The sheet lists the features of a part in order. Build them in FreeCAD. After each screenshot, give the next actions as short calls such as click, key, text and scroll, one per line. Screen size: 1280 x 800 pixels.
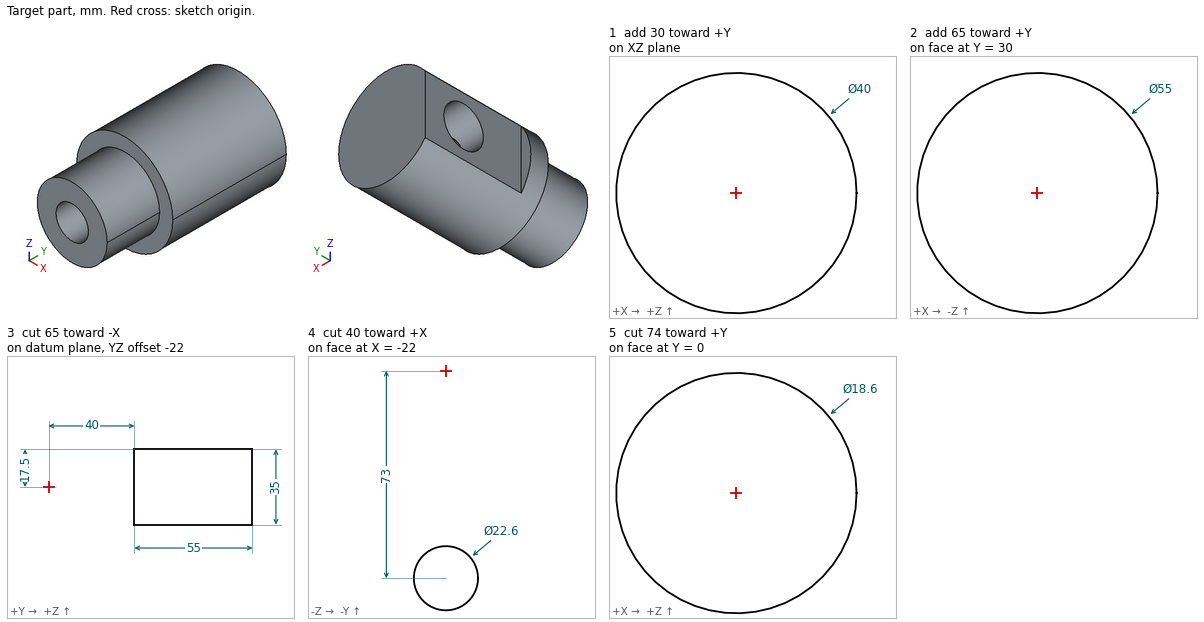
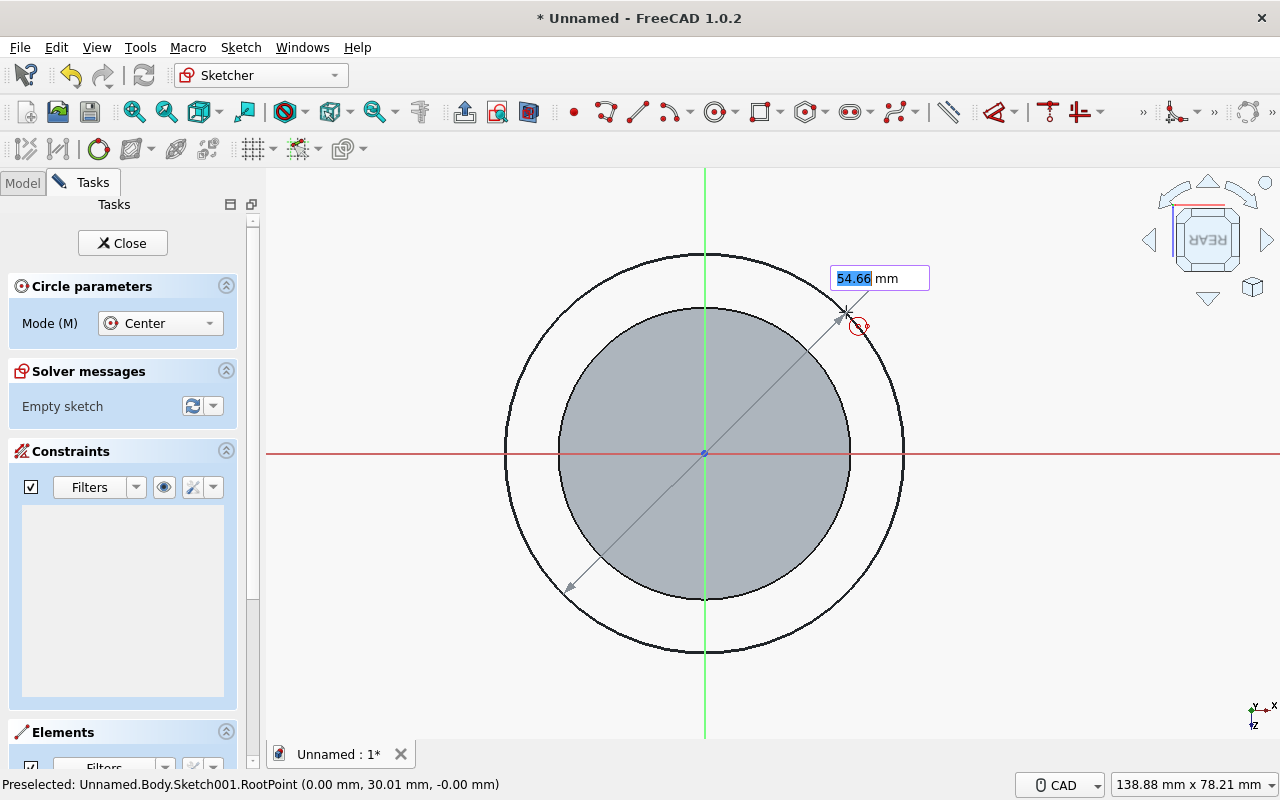
text(55)
key(Return)
key(Escape)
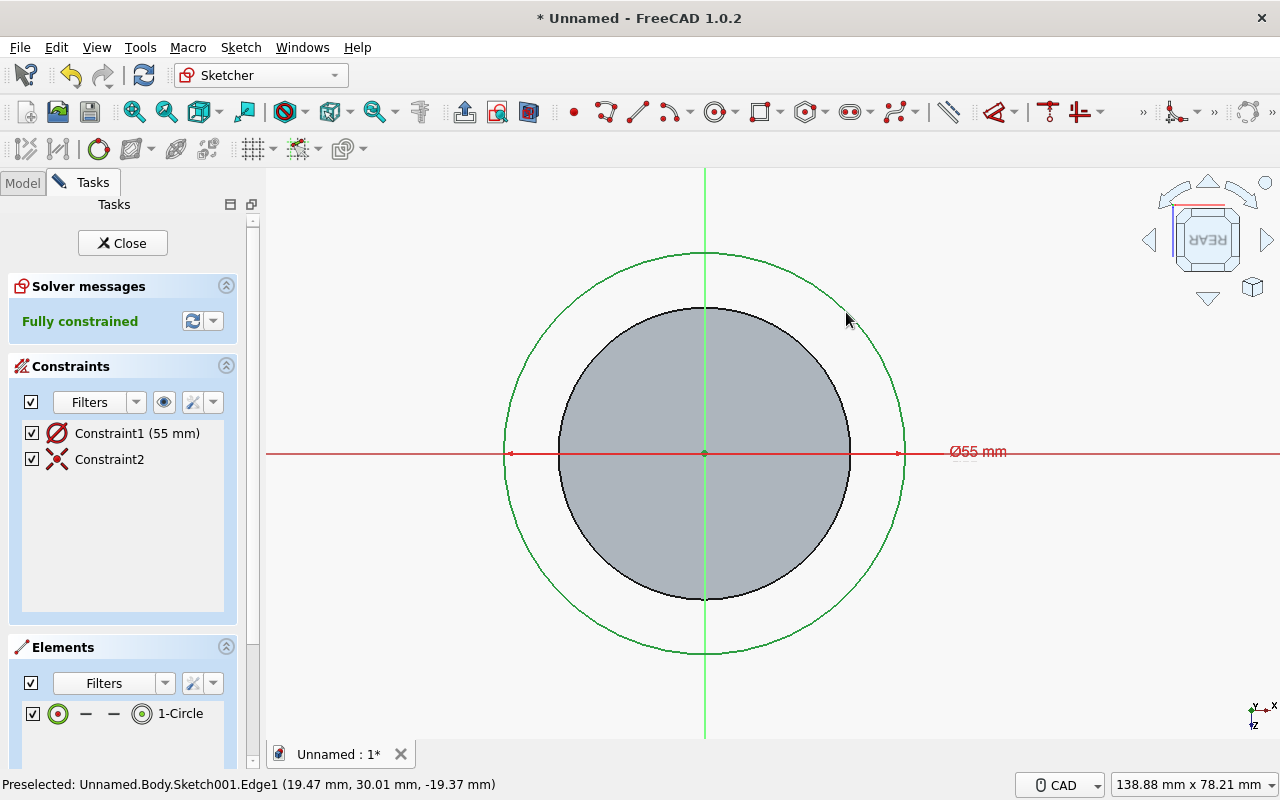
click(123, 243)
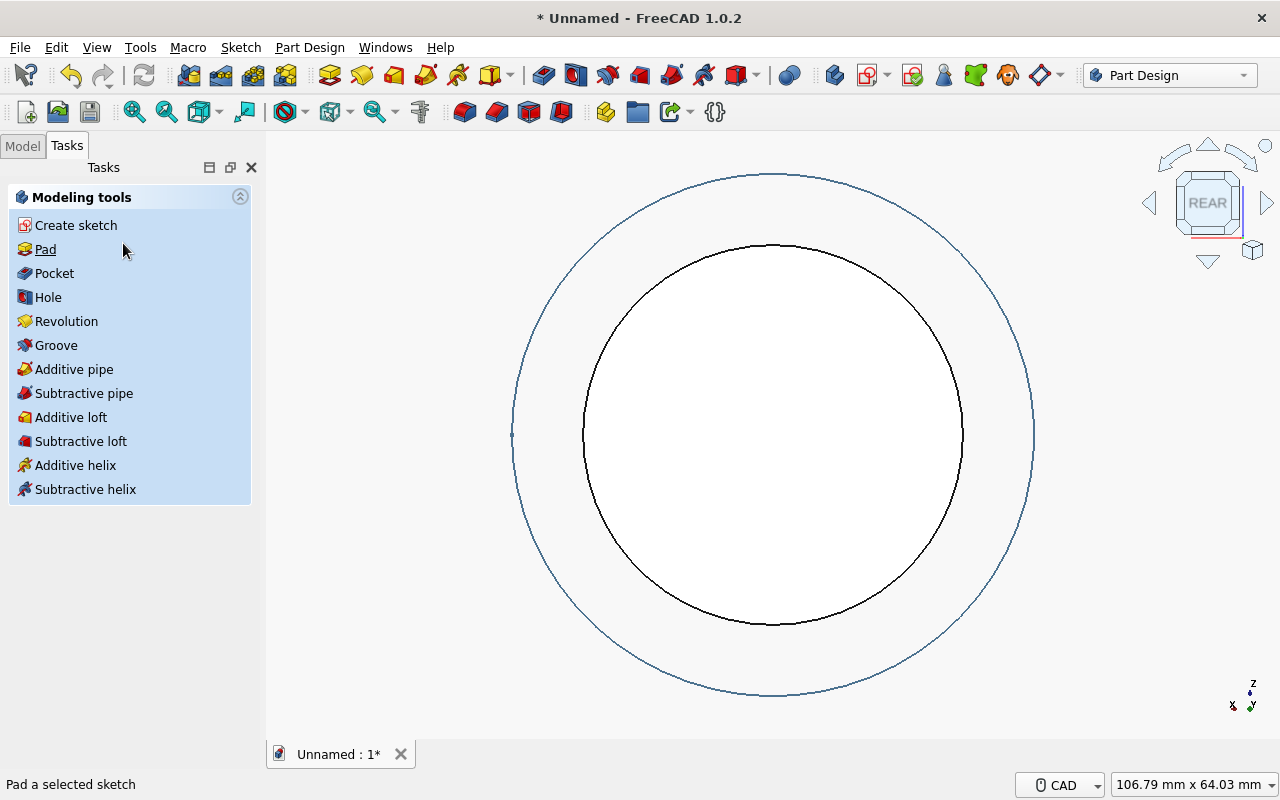
click(330, 76)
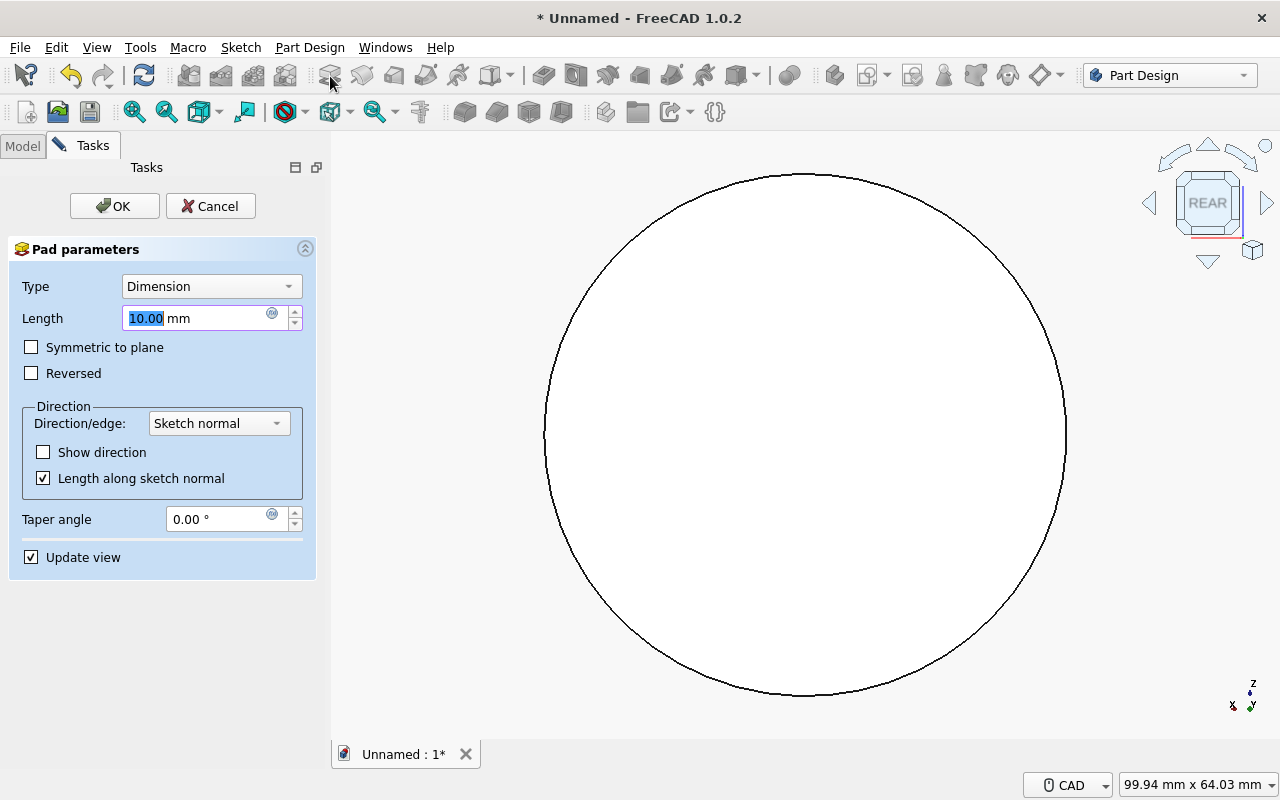
text(65)
key(Tab)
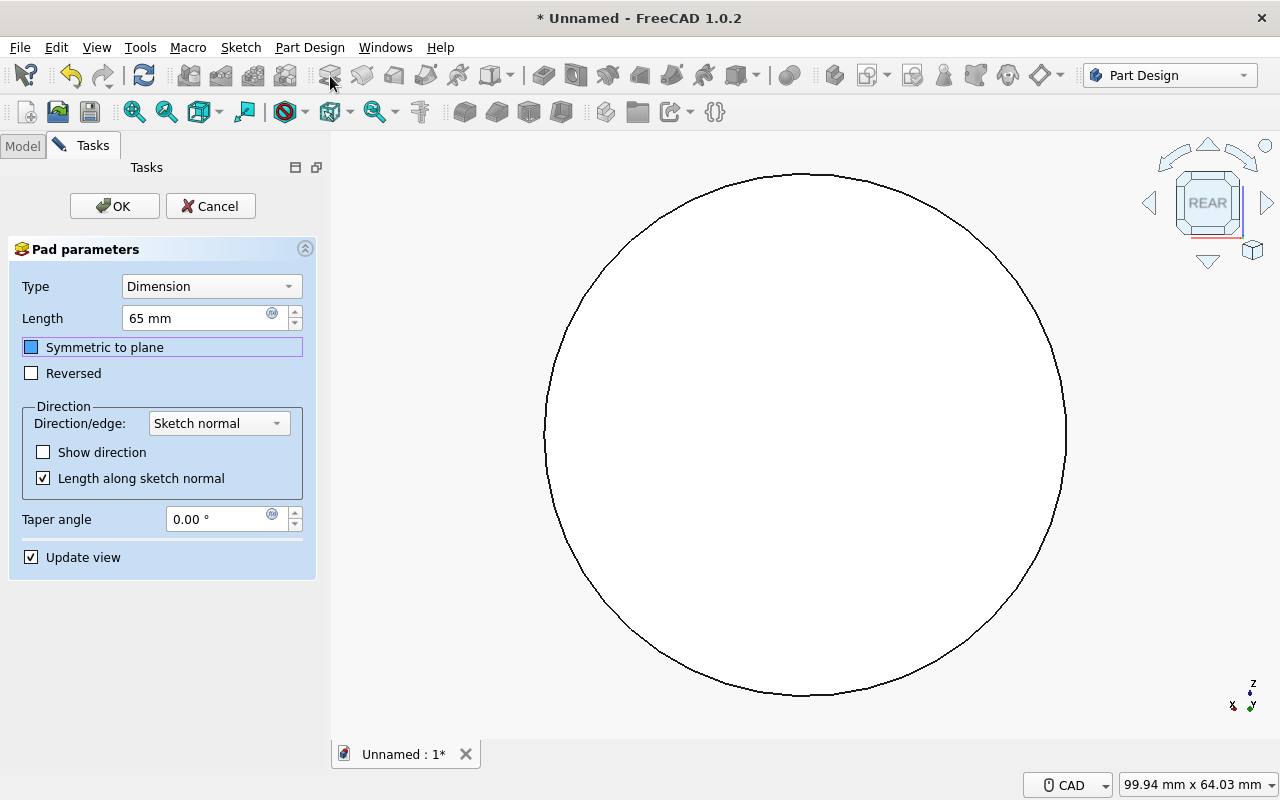
click(115, 206)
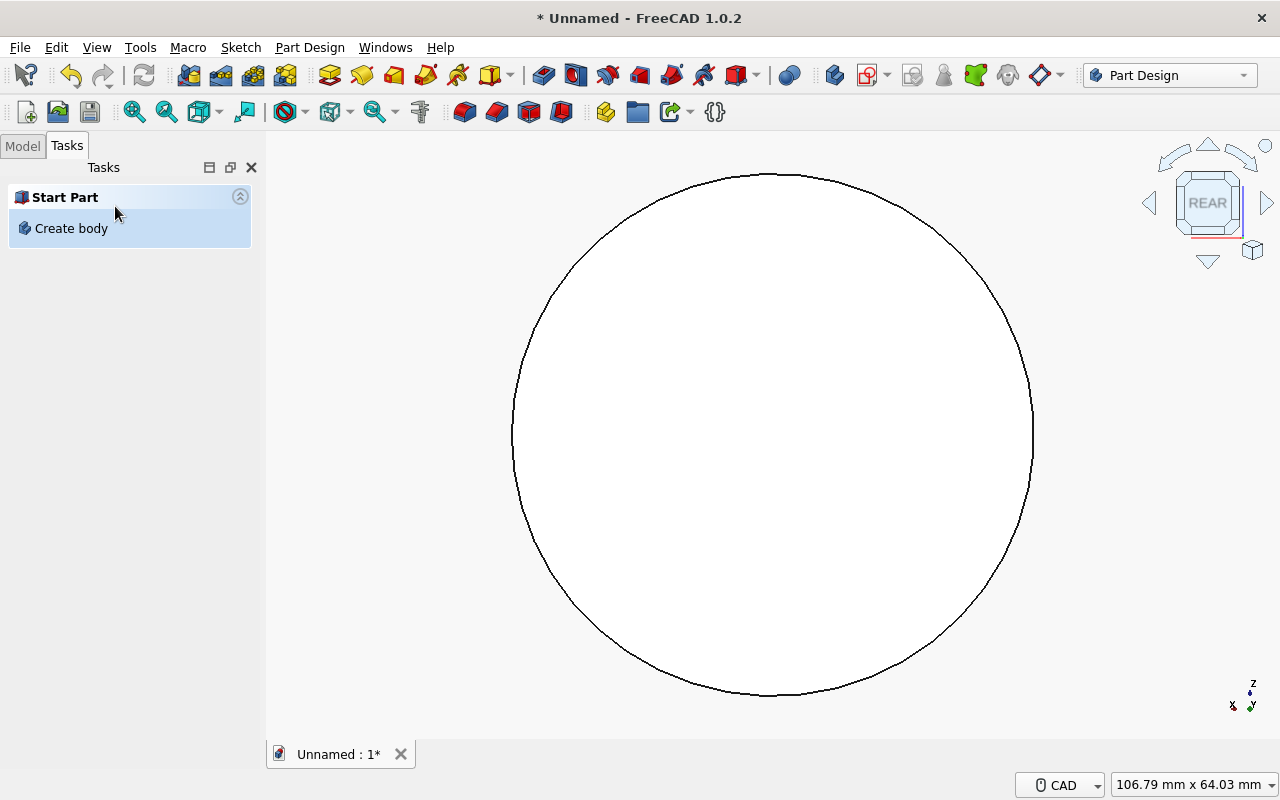
click(23, 145)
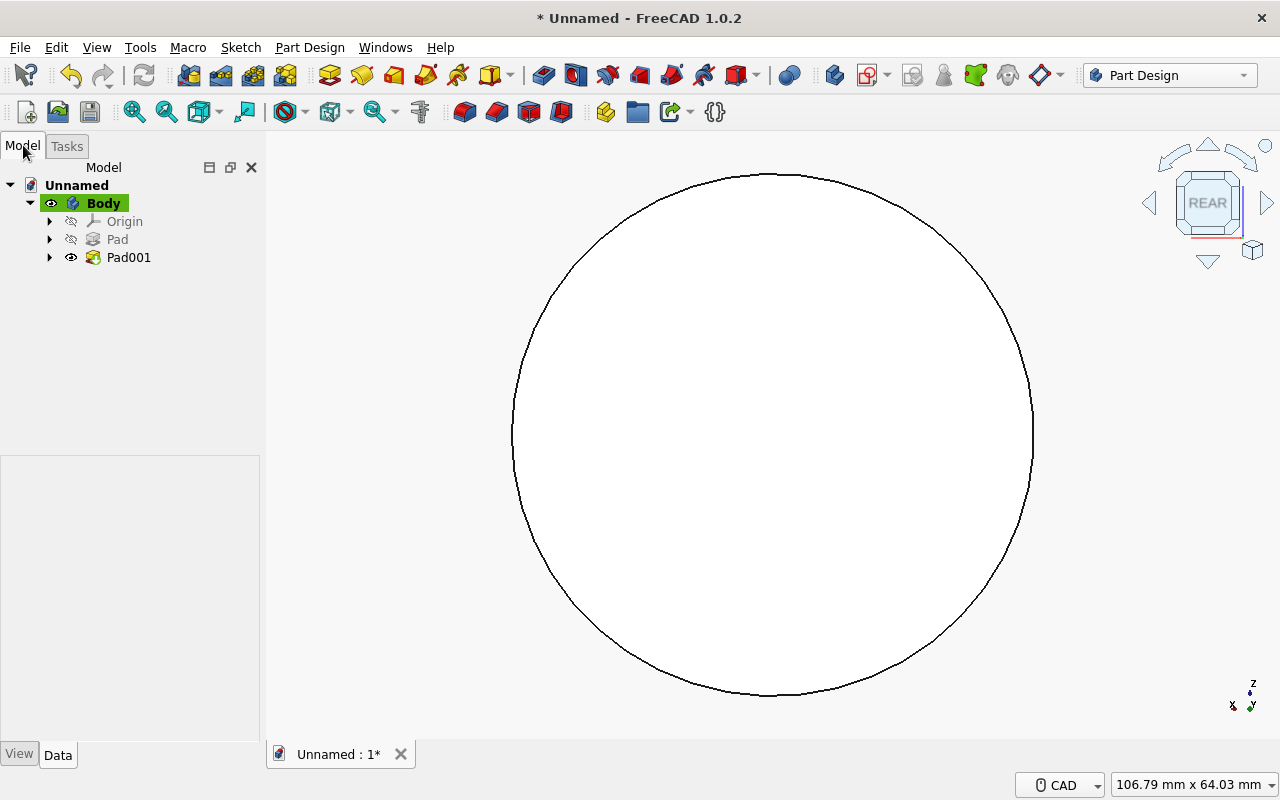
click(50, 221)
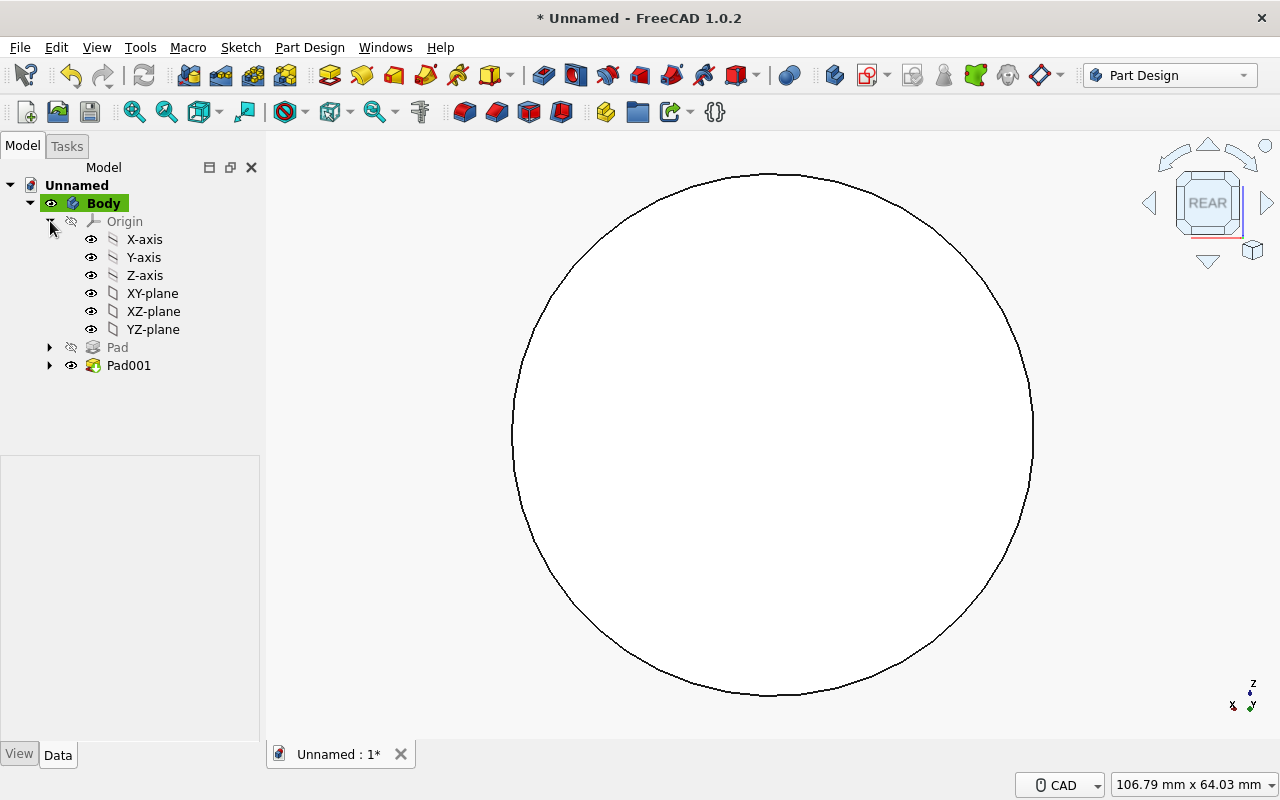
click(136, 329)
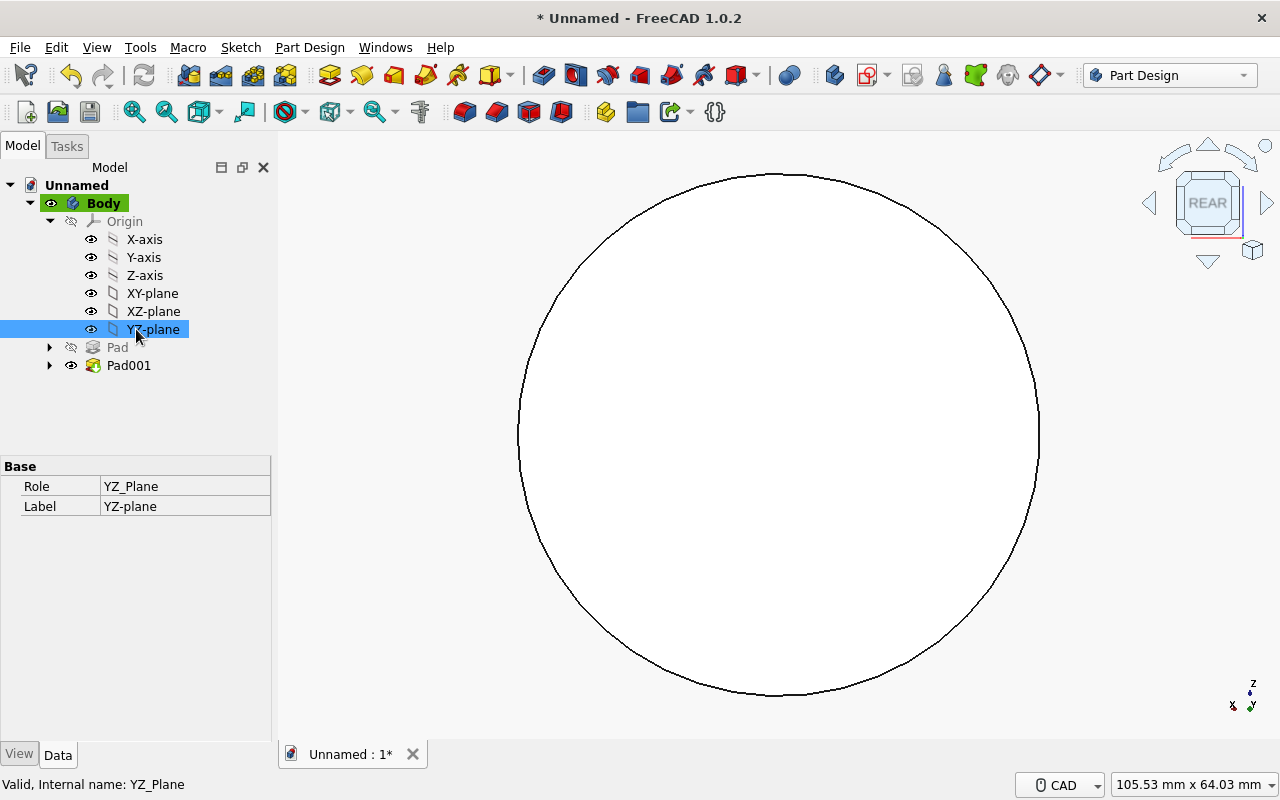
click(1040, 76)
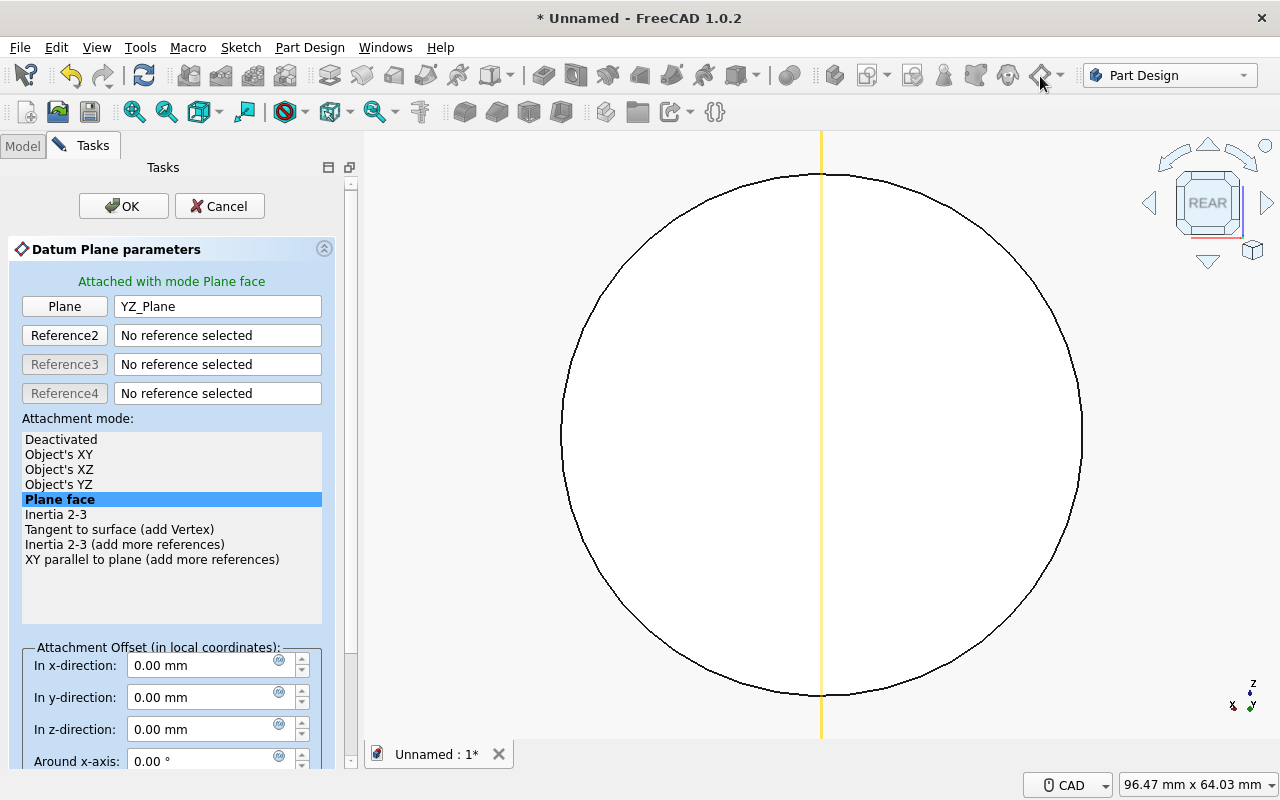
triple_click(210, 729)